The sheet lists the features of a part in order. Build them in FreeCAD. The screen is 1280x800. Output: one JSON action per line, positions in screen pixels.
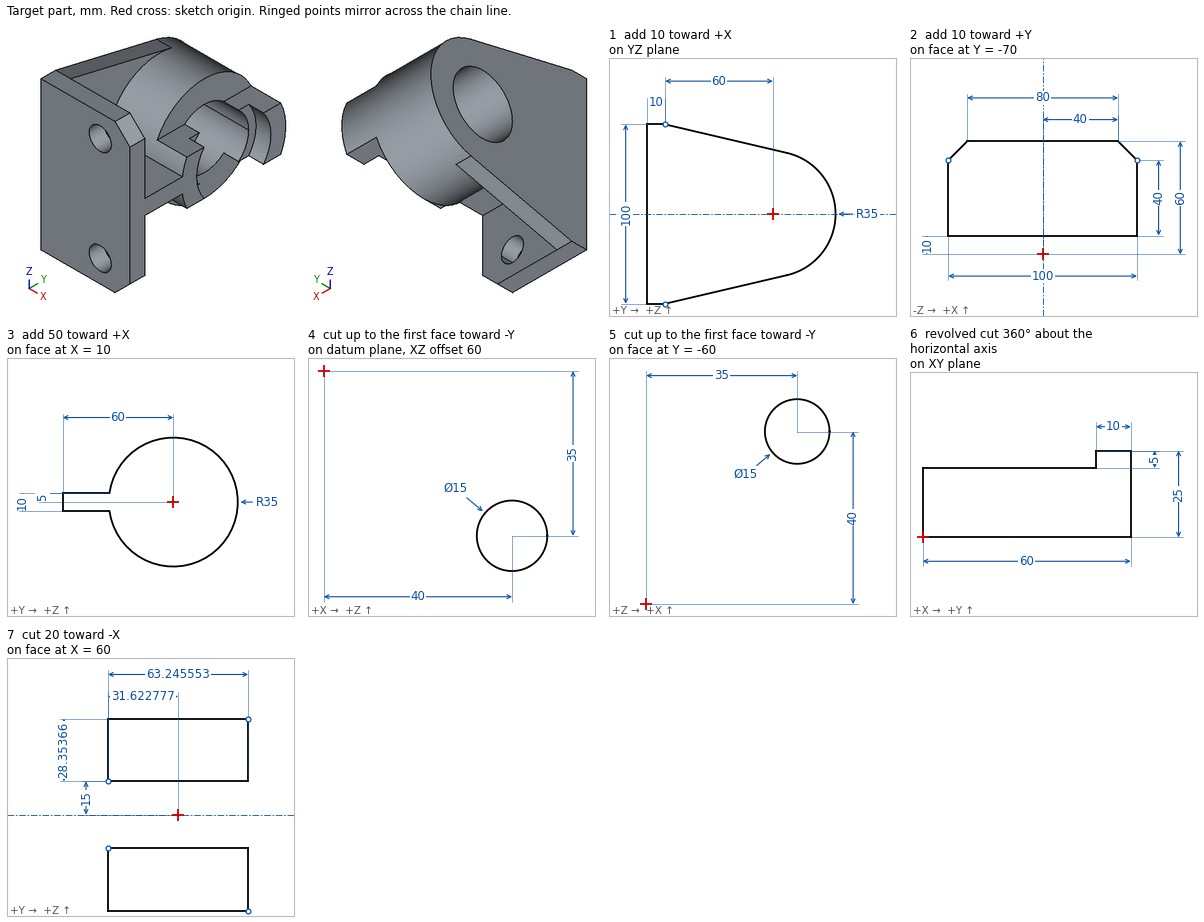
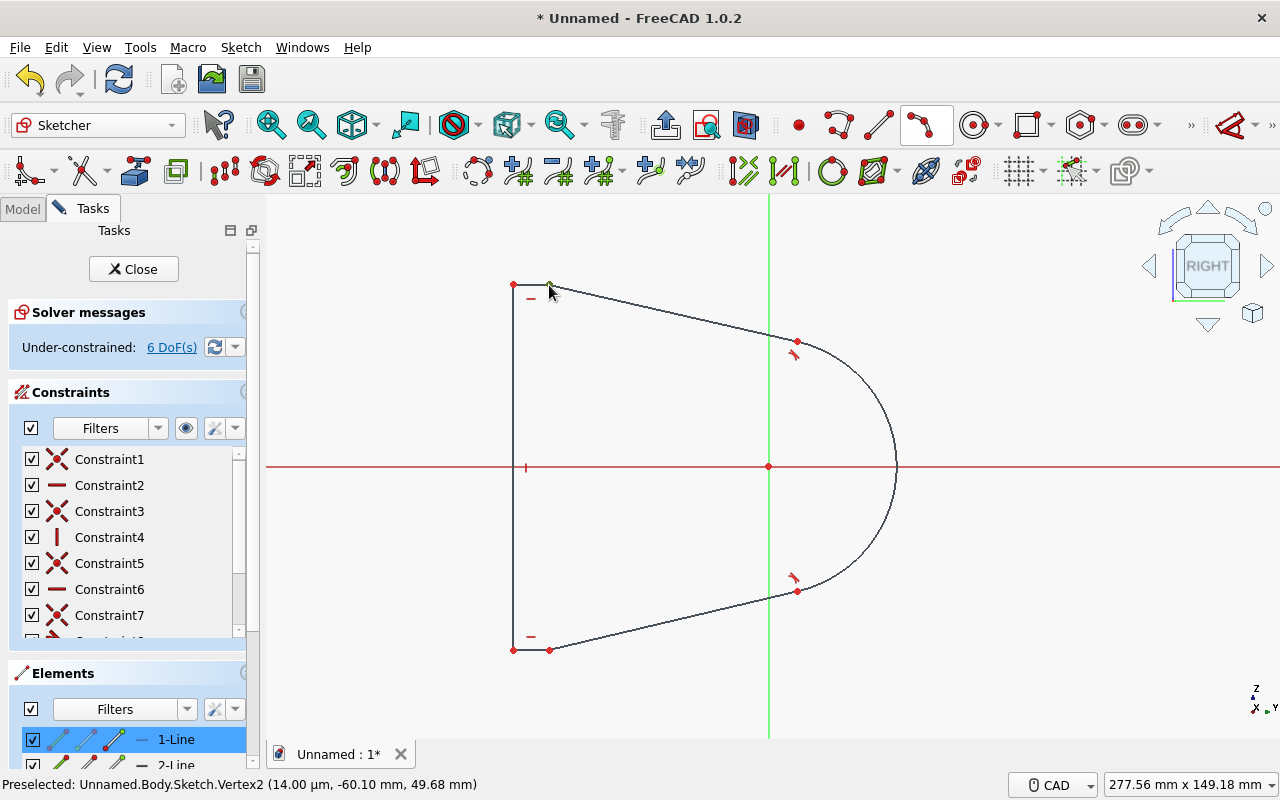
{"action": "left_click", "coordinate": [549, 650]}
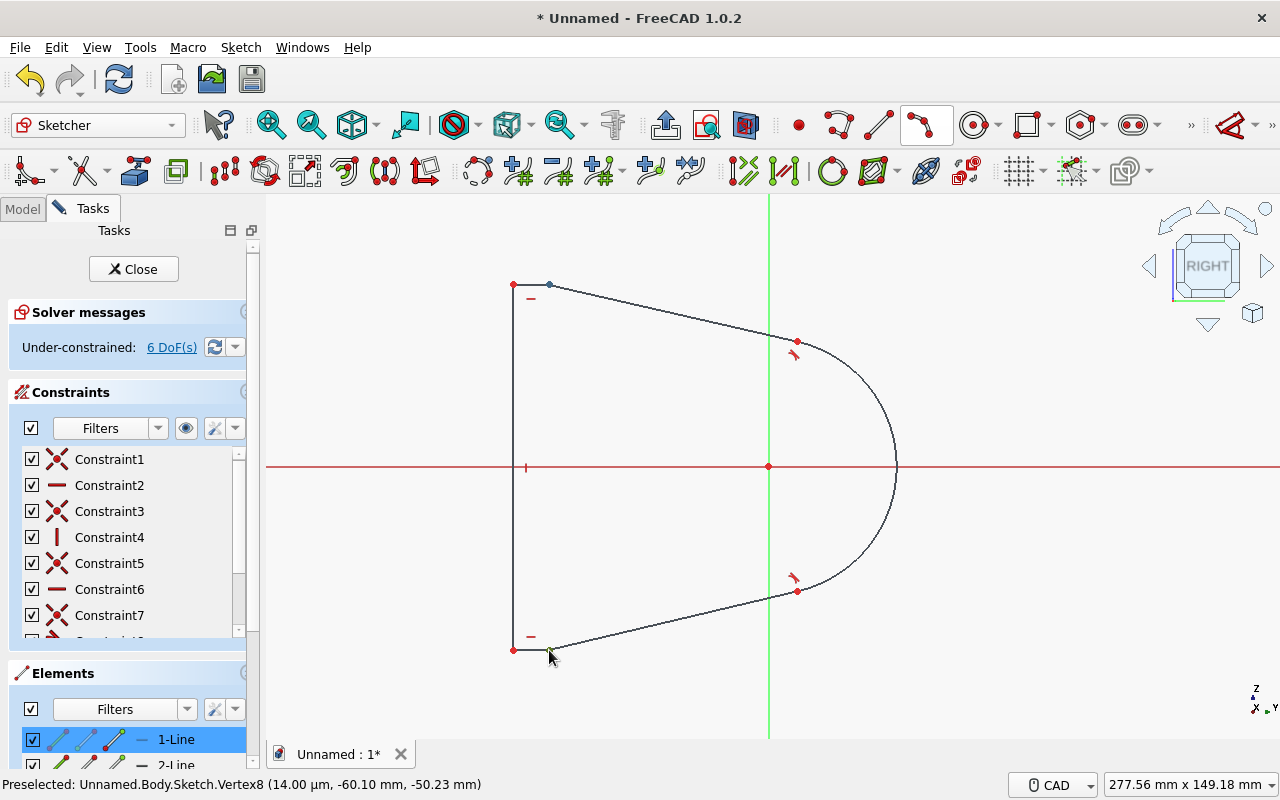
{"action": "left_click", "coordinate": [353, 466]}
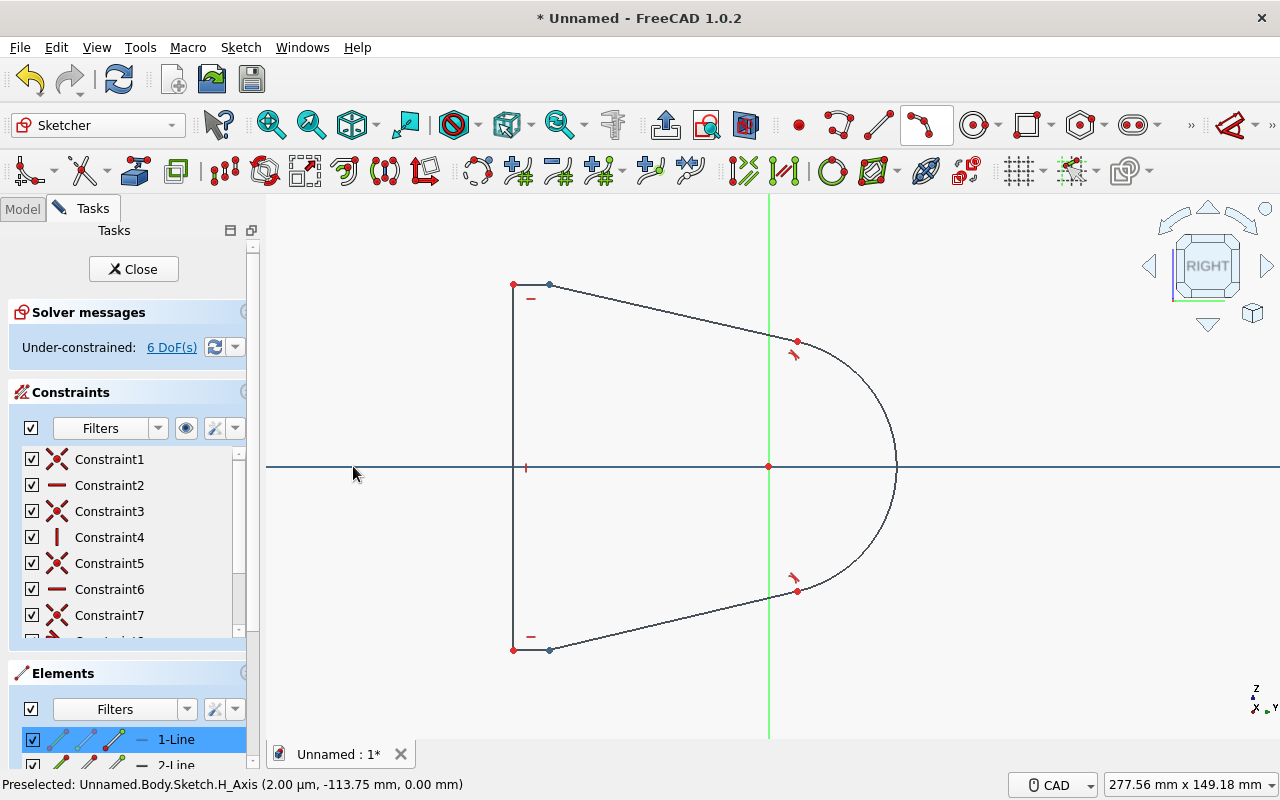
{"action": "key", "text": "s"}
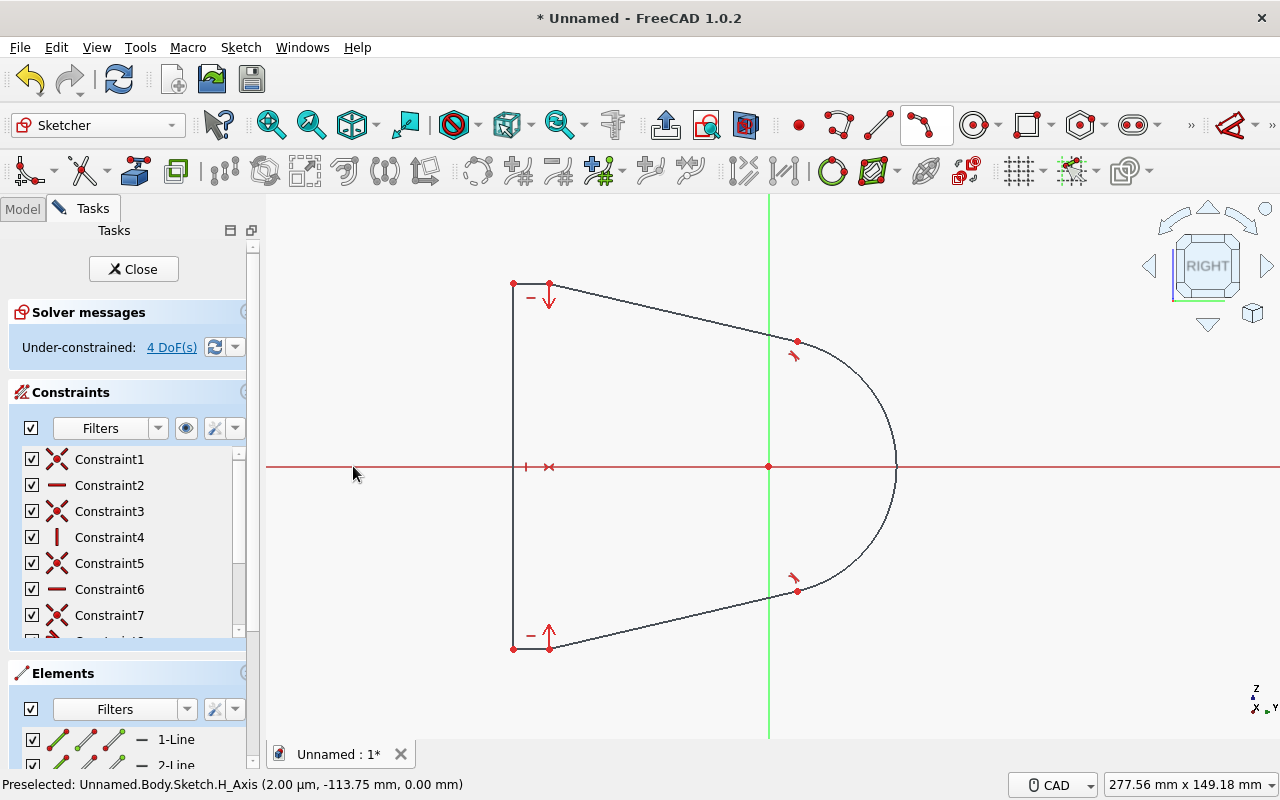
{"action": "key", "text": "d"}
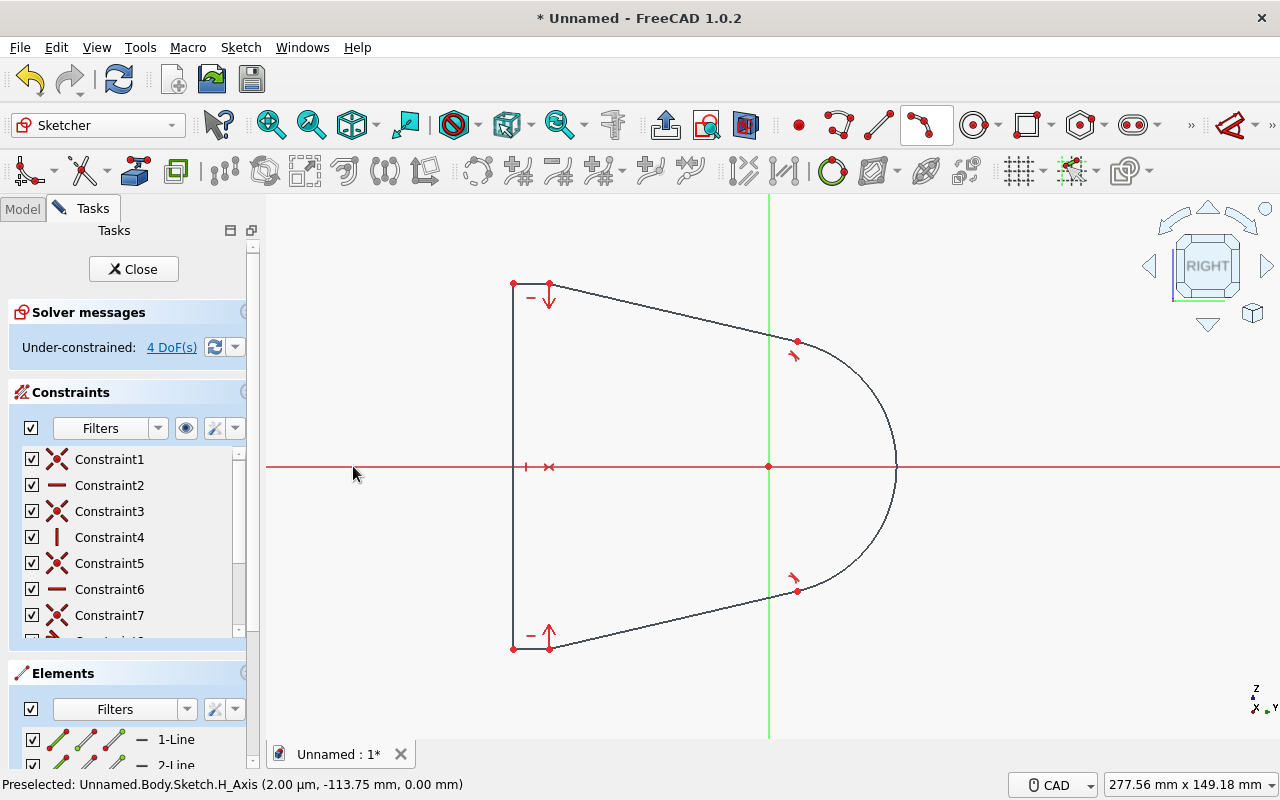
{"action": "left_click", "coordinate": [879, 532]}
{"action": "left_click", "coordinate": [907, 548]}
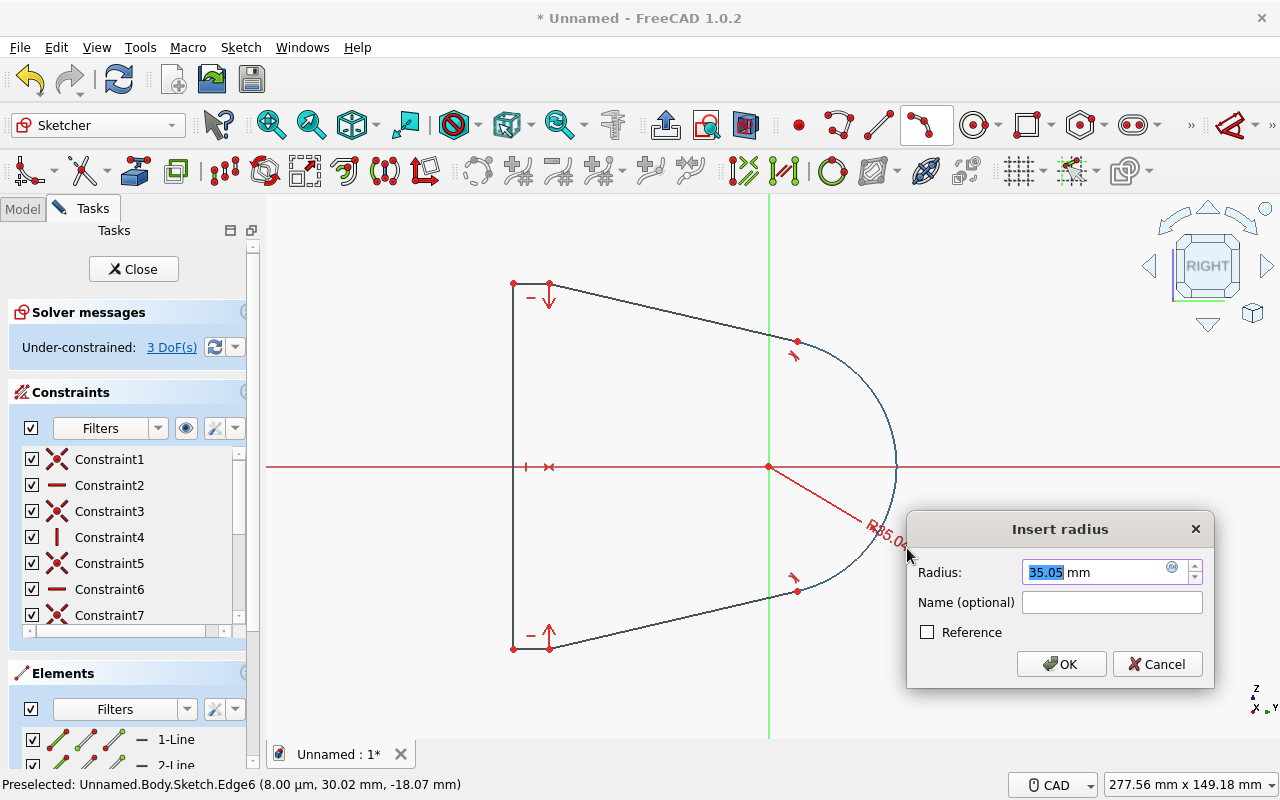
{"action": "type", "text": "35"}
{"action": "key", "text": "Return"}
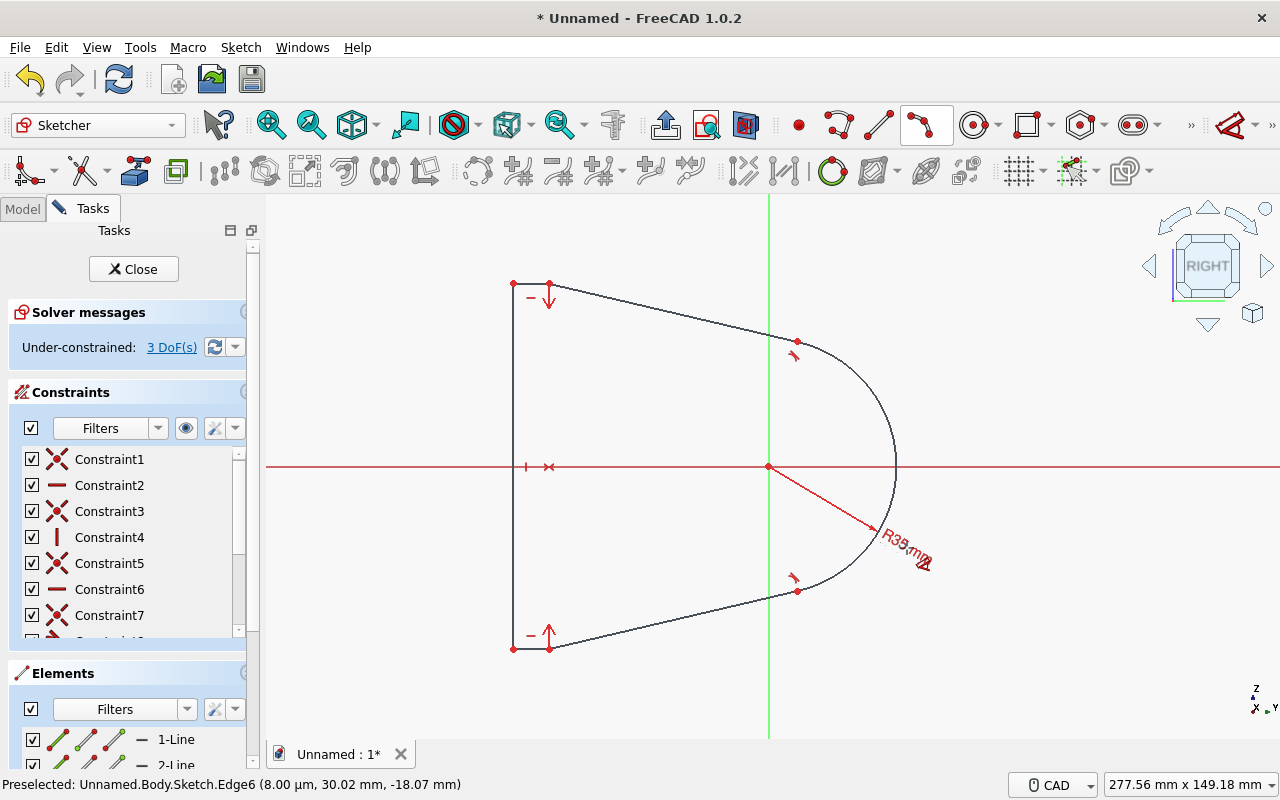
{"action": "scroll", "coordinate": [538, 284], "scroll_direction": "up", "scroll_amount": 2}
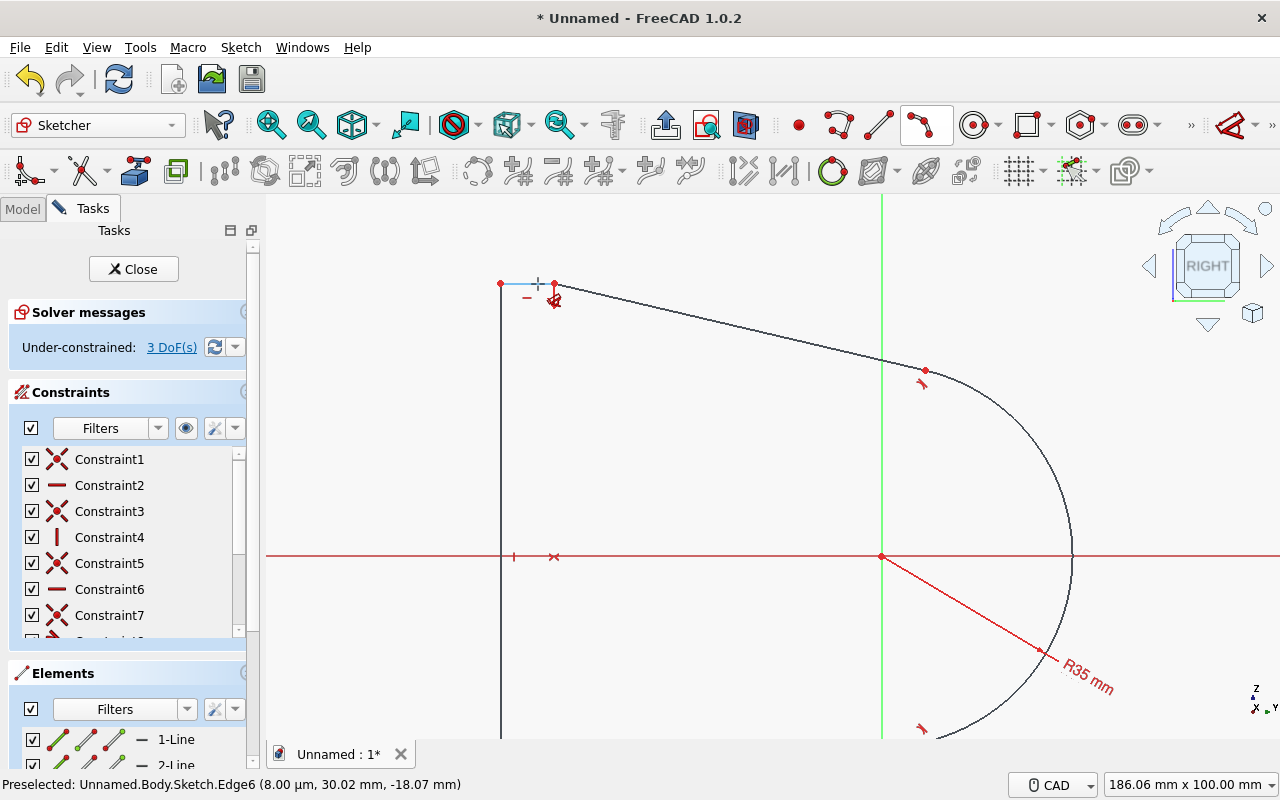
{"action": "left_click", "coordinate": [538, 284]}
{"action": "left_click", "coordinate": [527, 250]}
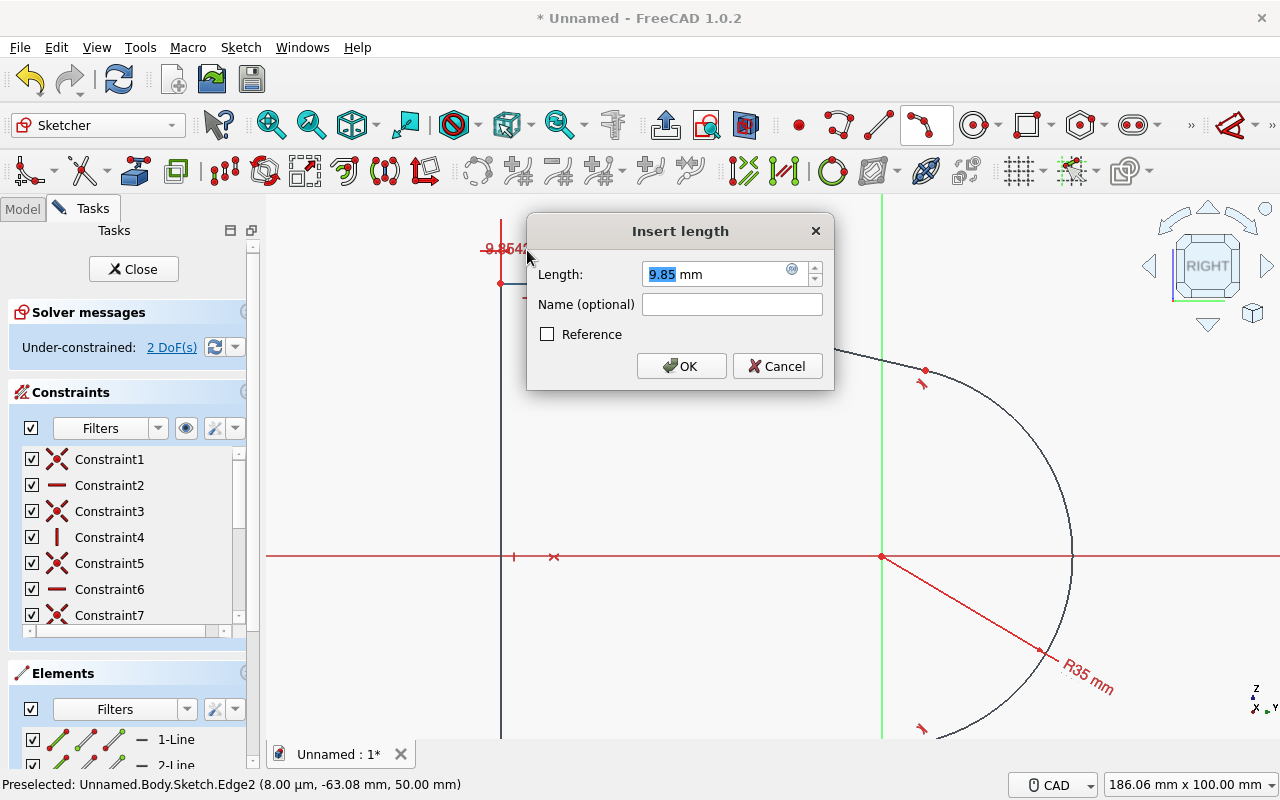
{"action": "type", "text": "10"}
{"action": "key", "text": "Return"}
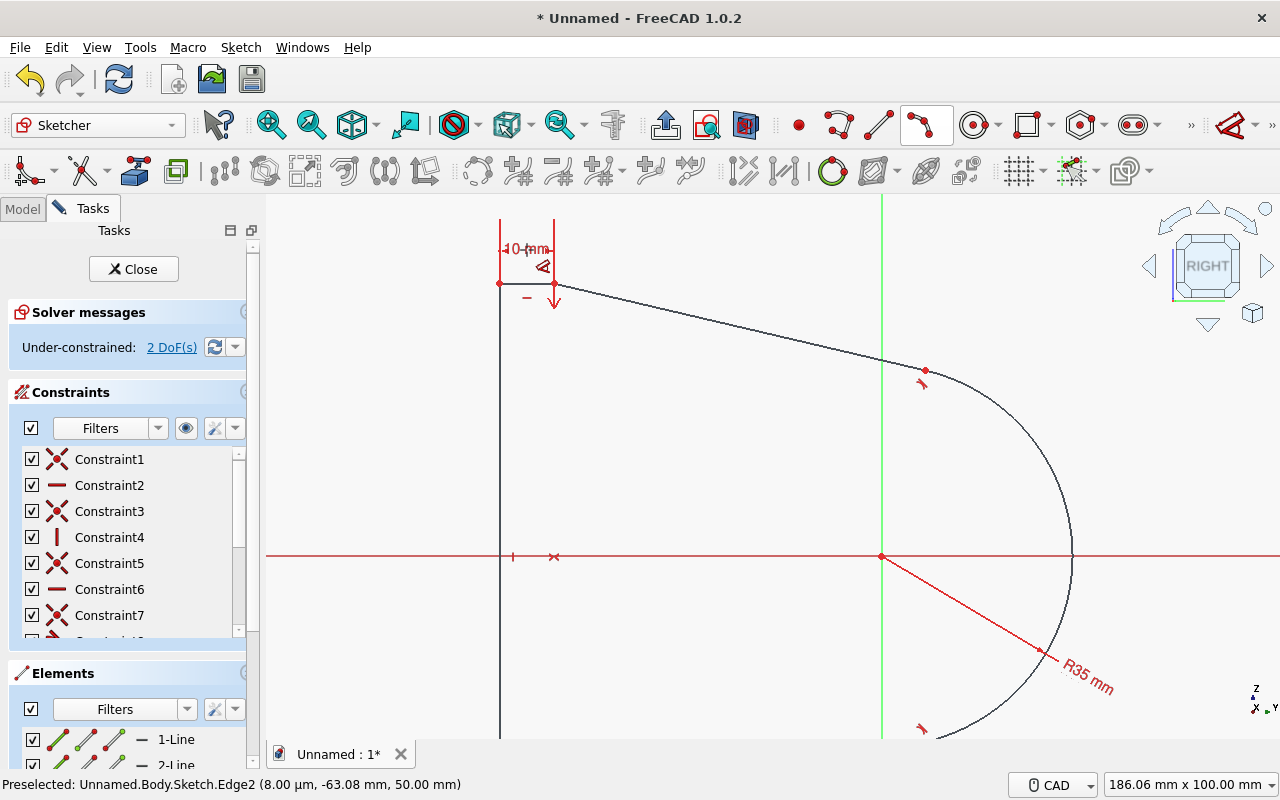
{"action": "left_click", "coordinate": [500, 447]}
{"action": "left_click", "coordinate": [466, 497]}